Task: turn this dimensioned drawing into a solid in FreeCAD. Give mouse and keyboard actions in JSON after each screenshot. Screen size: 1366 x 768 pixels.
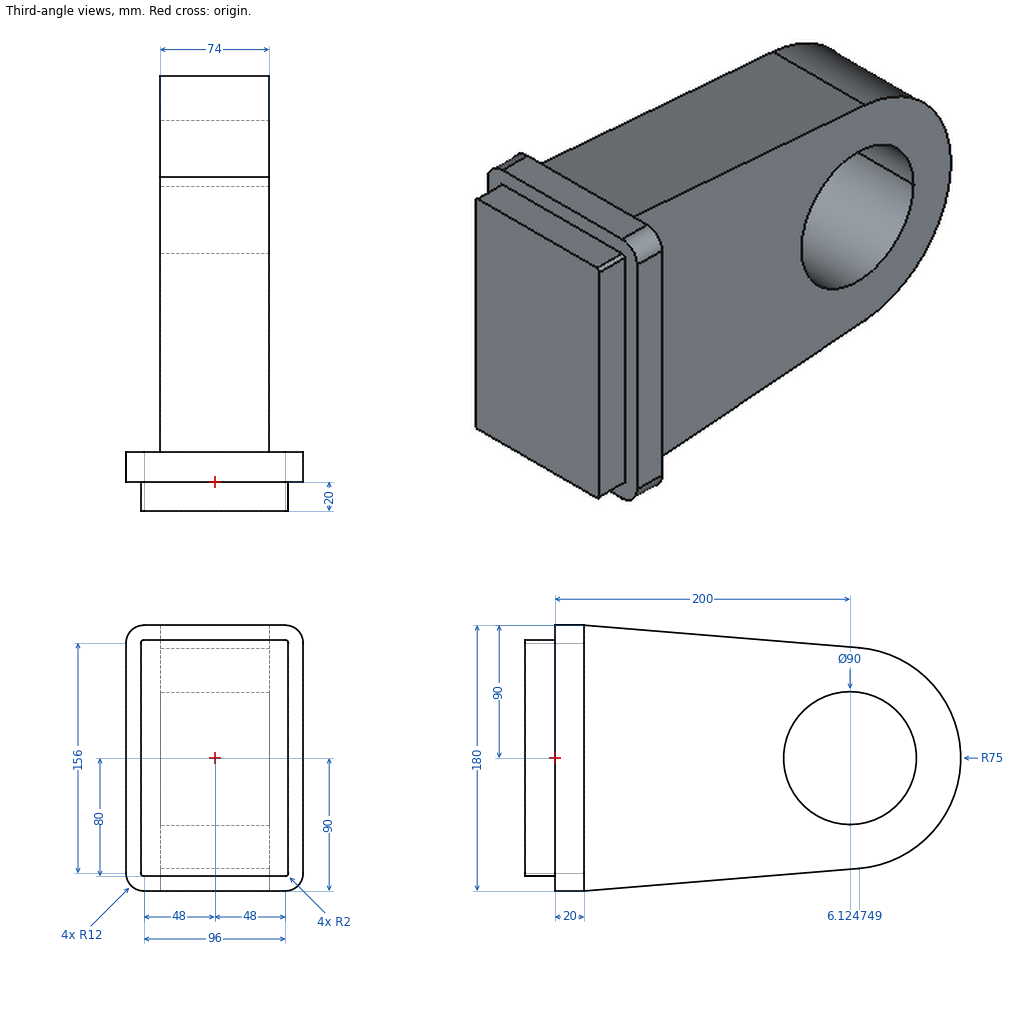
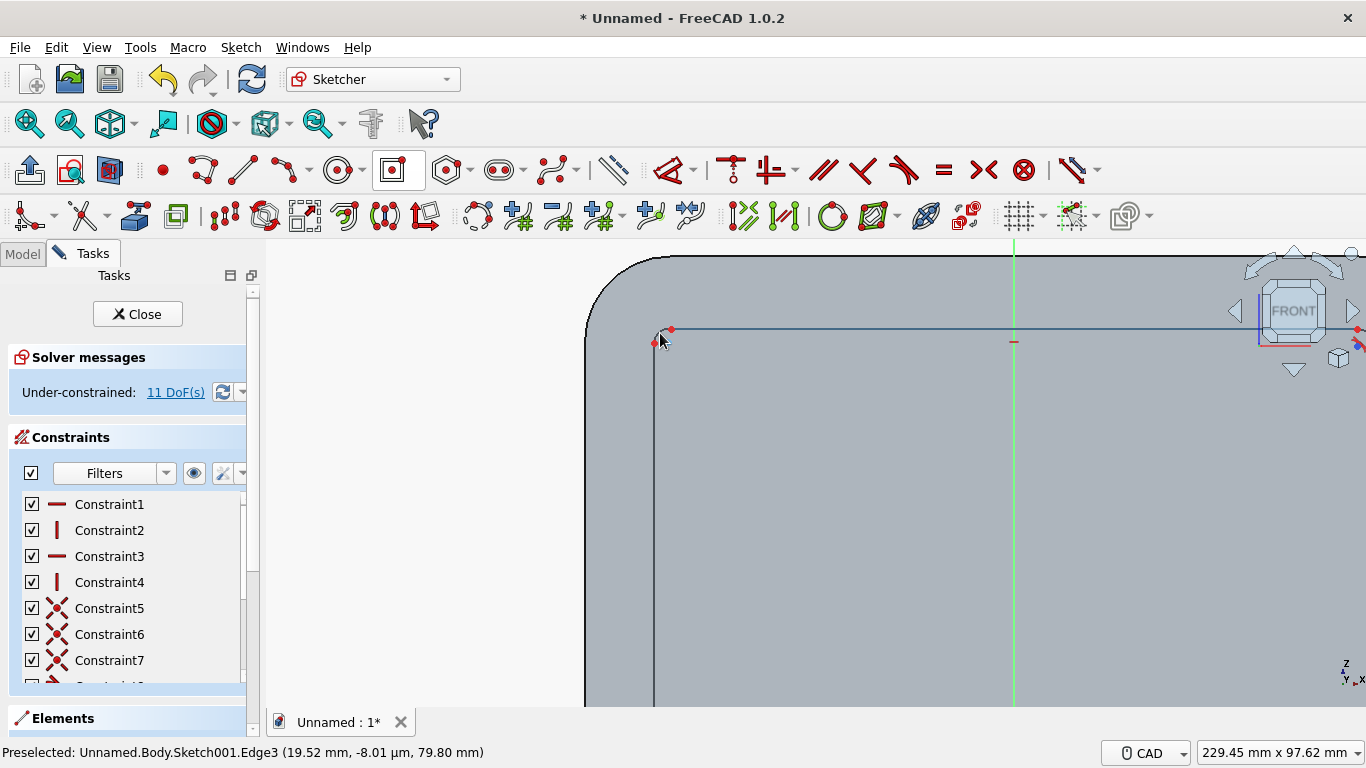
{"action": "left_click", "coordinate": [659, 332]}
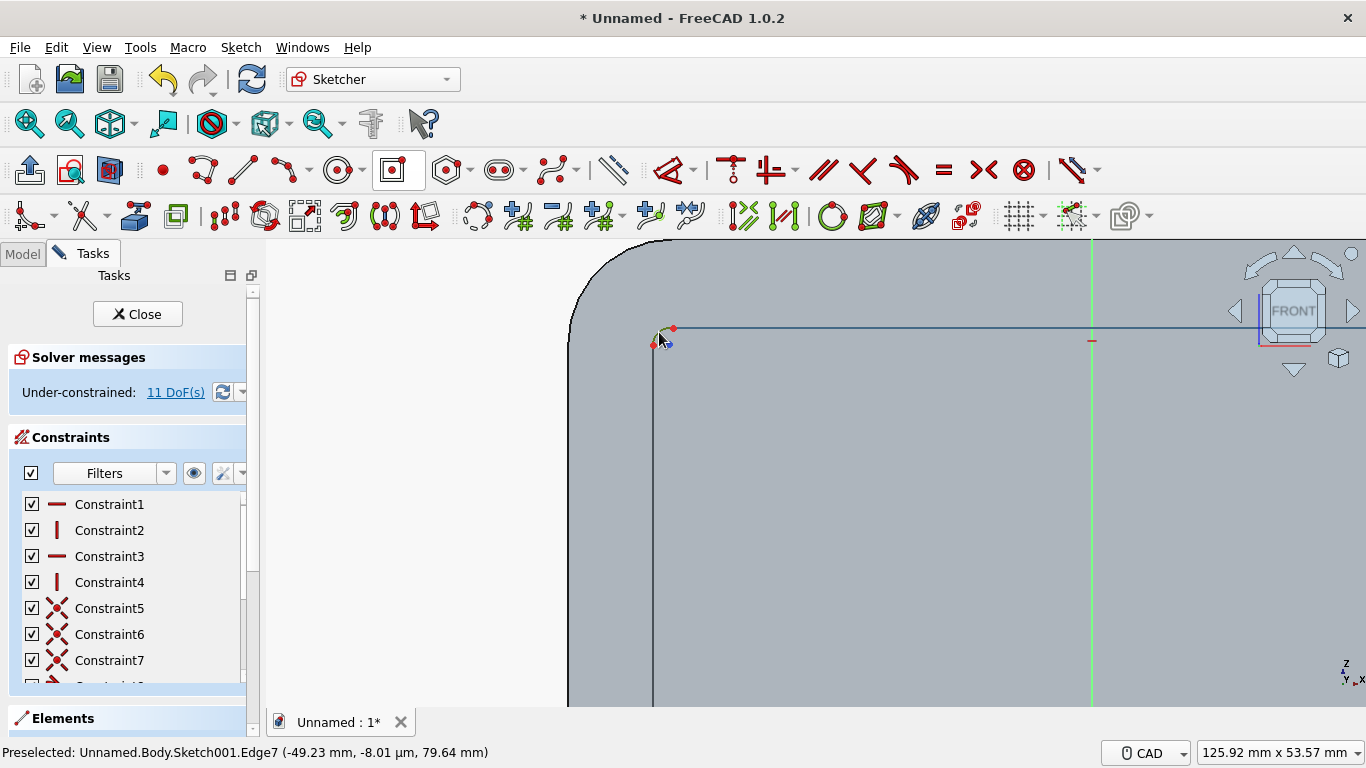
{"action": "left_click", "coordinate": [904, 170]}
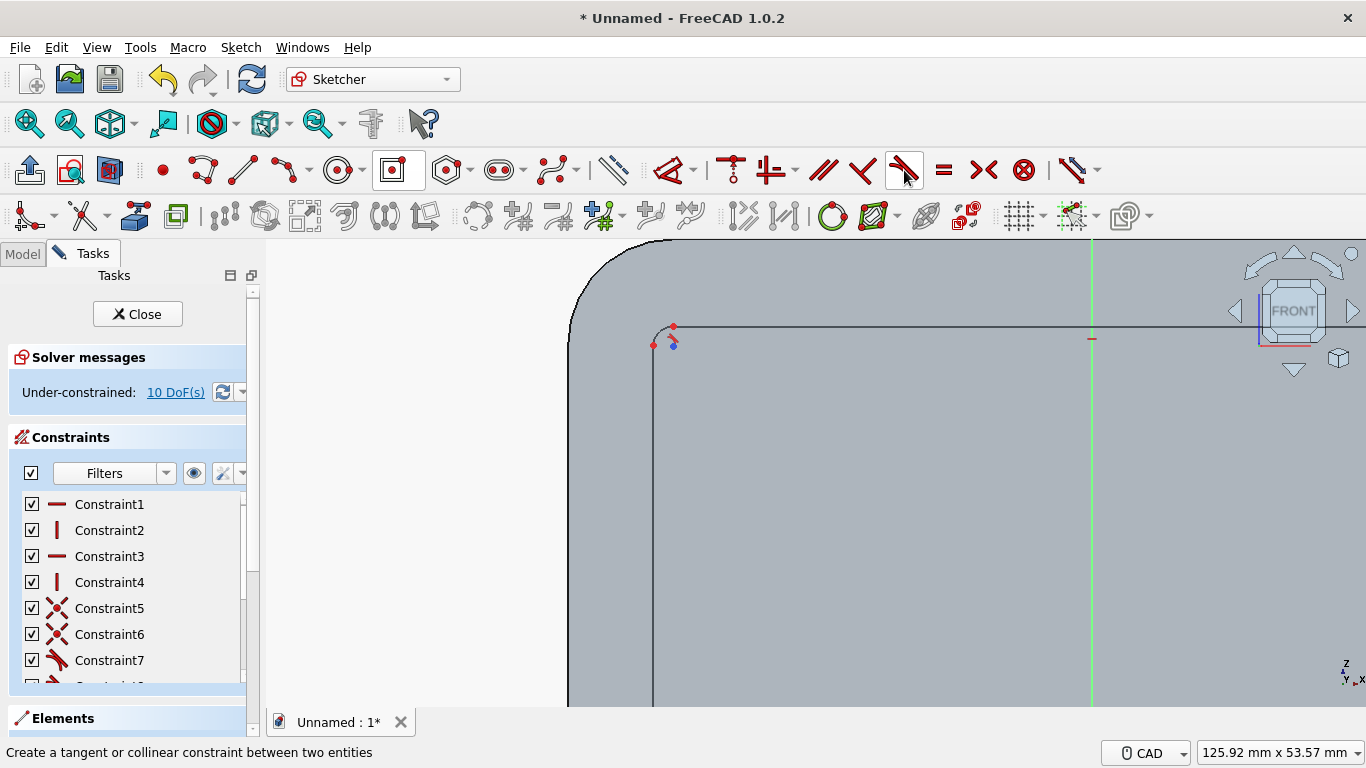
{"action": "scroll", "coordinate": [660, 333], "scroll_direction": "down", "scroll_amount": 8}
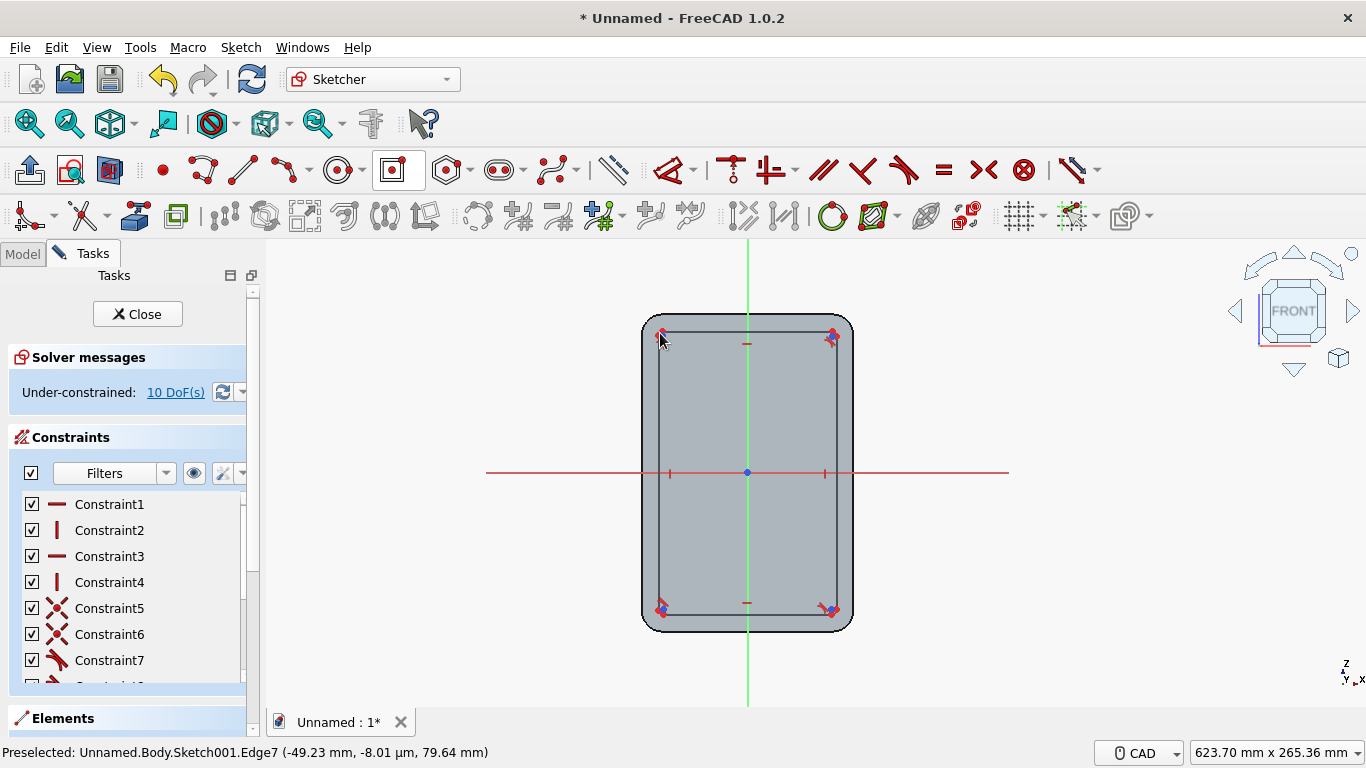
{"action": "left_click", "coordinate": [659, 391]}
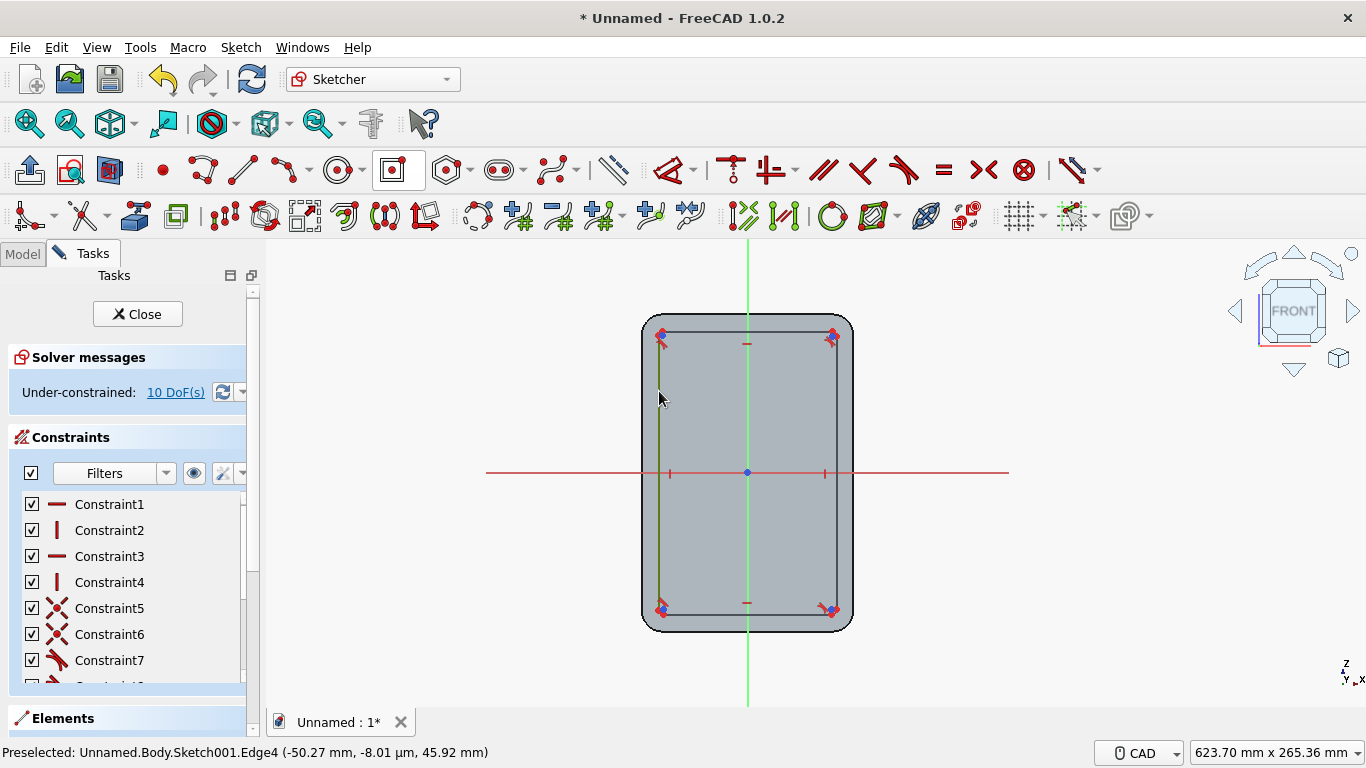
{"action": "scroll", "coordinate": [660, 333], "scroll_direction": "up", "scroll_amount": 8}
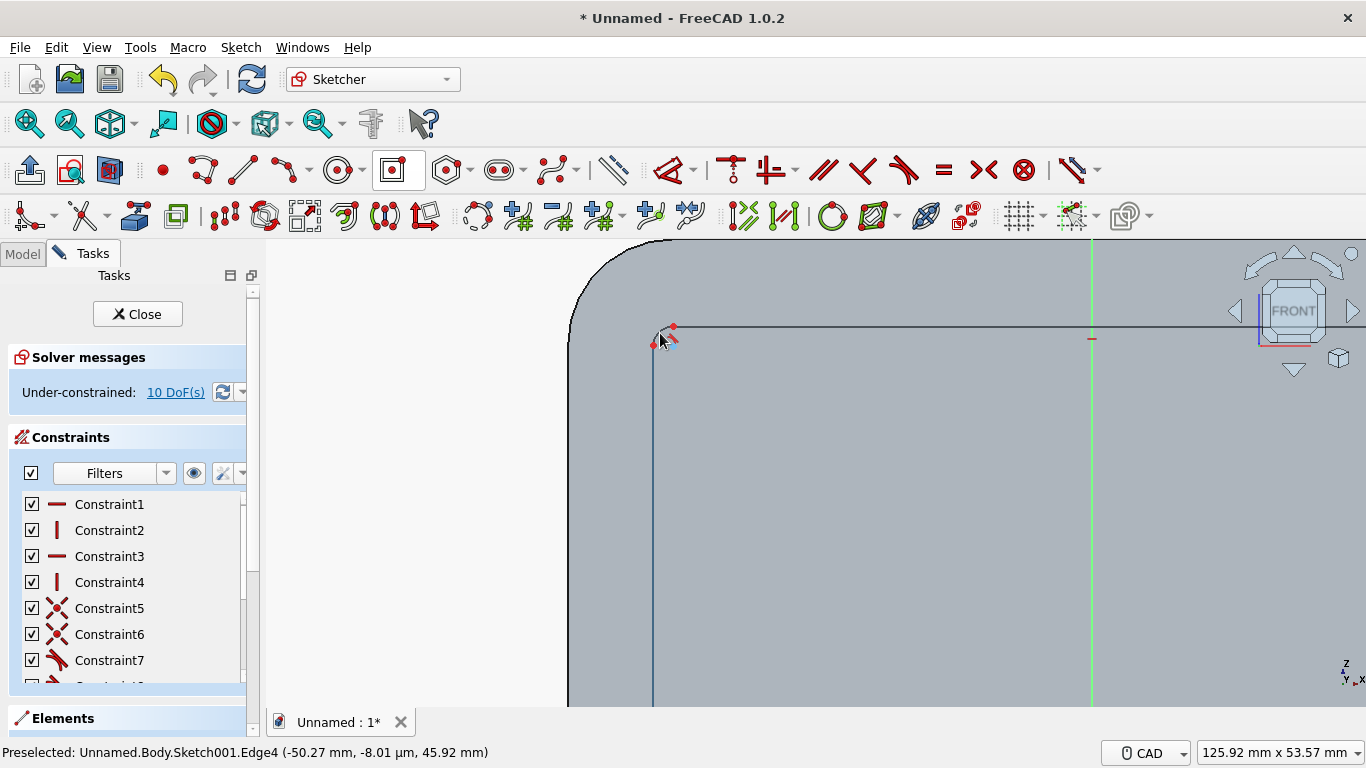
{"action": "left_click", "coordinate": [660, 332]}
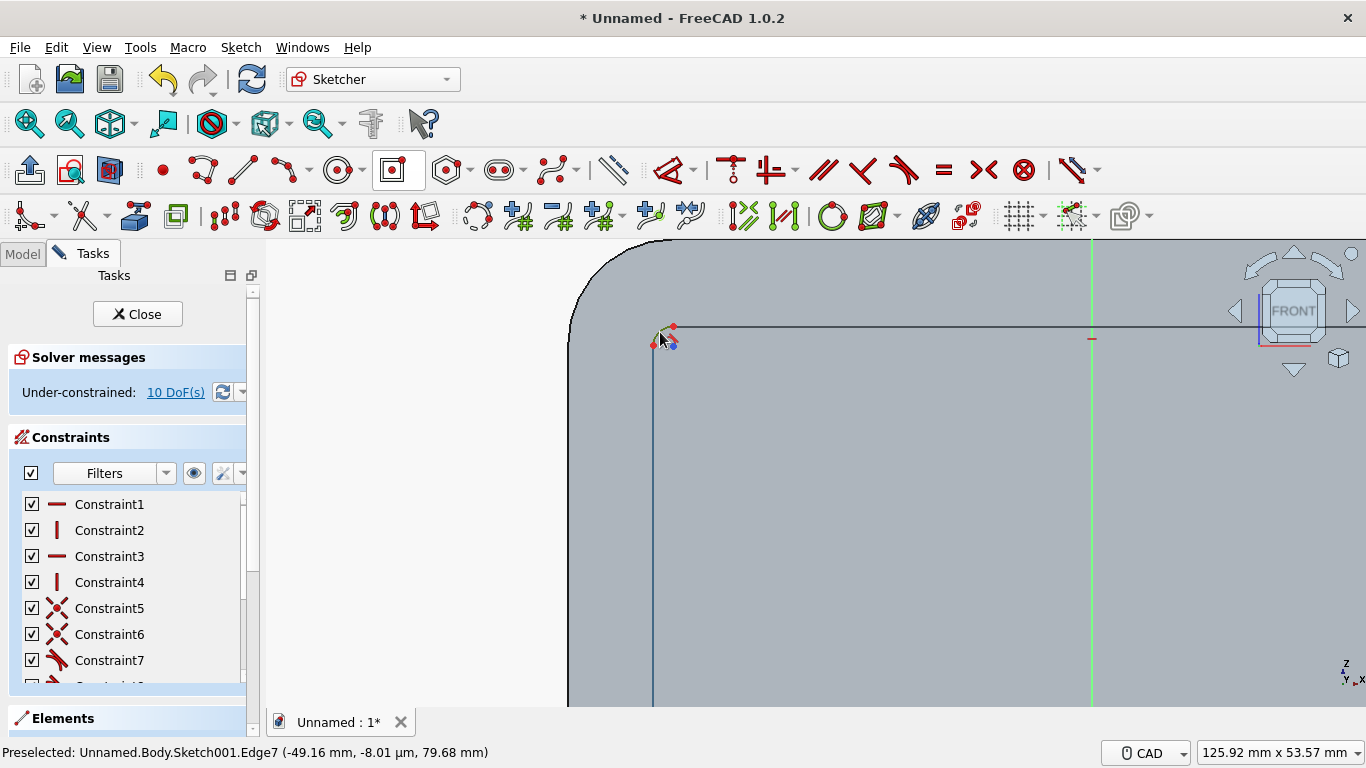
{"action": "key", "text": "t"}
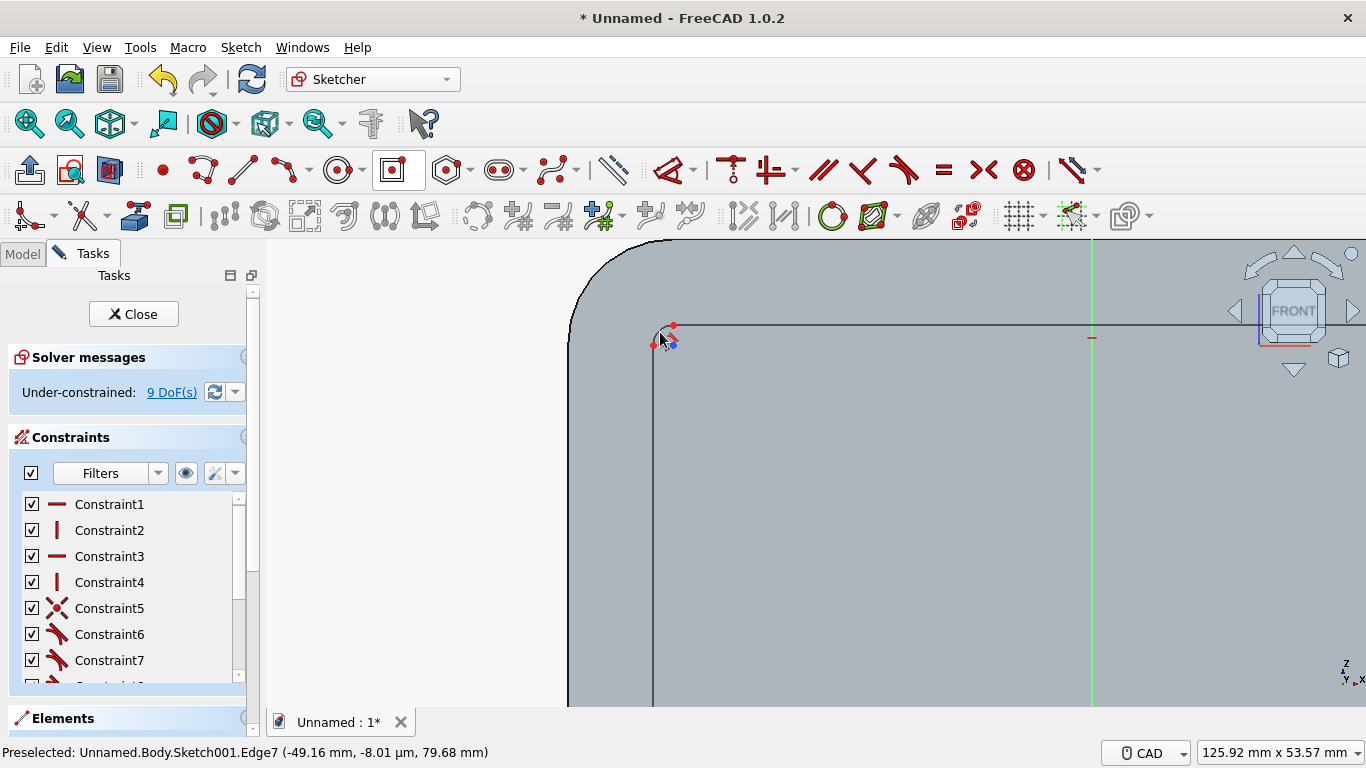
{"action": "scroll", "coordinate": [660, 333], "scroll_direction": "down", "scroll_amount": 8}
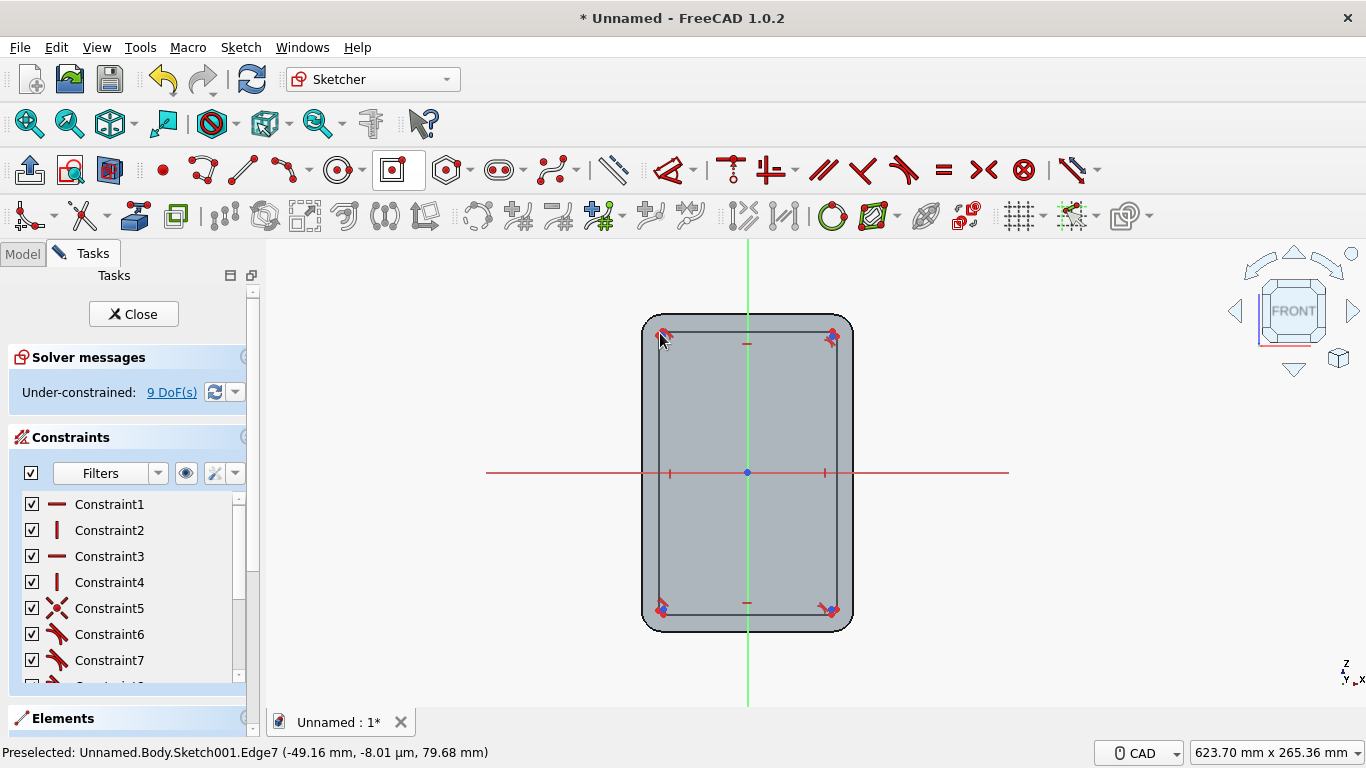
{"action": "left_click", "coordinate": [659, 391]}